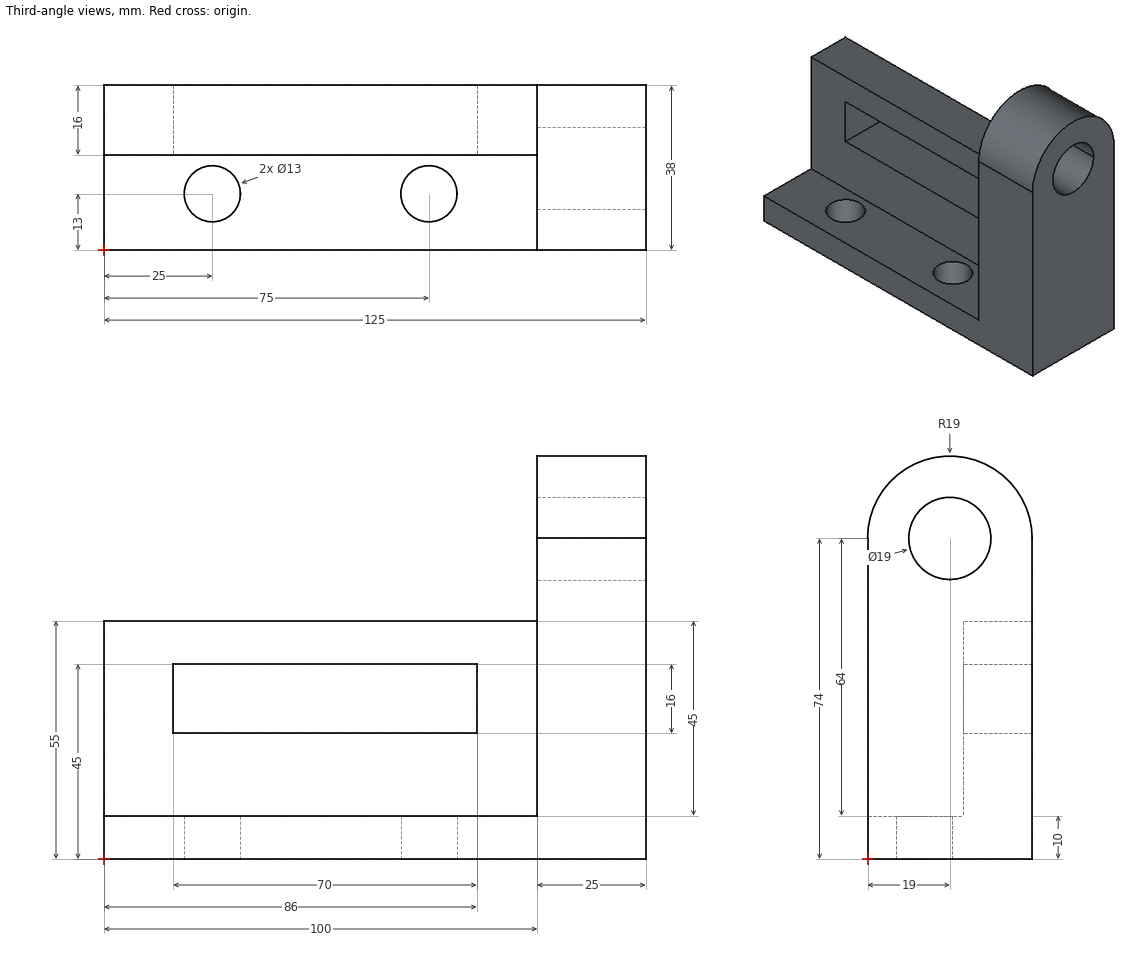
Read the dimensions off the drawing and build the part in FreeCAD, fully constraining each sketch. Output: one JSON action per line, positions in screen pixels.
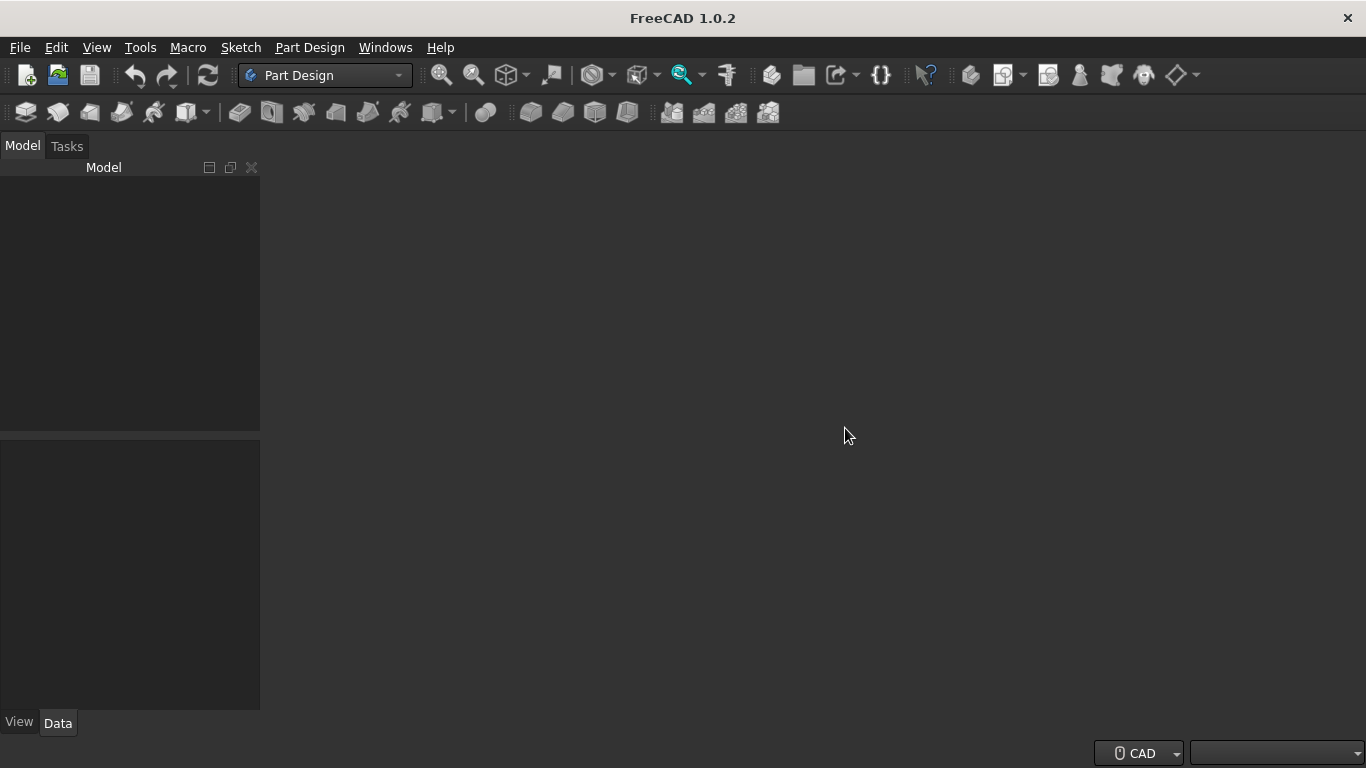
{"action": "left_click", "coordinate": [26, 76]}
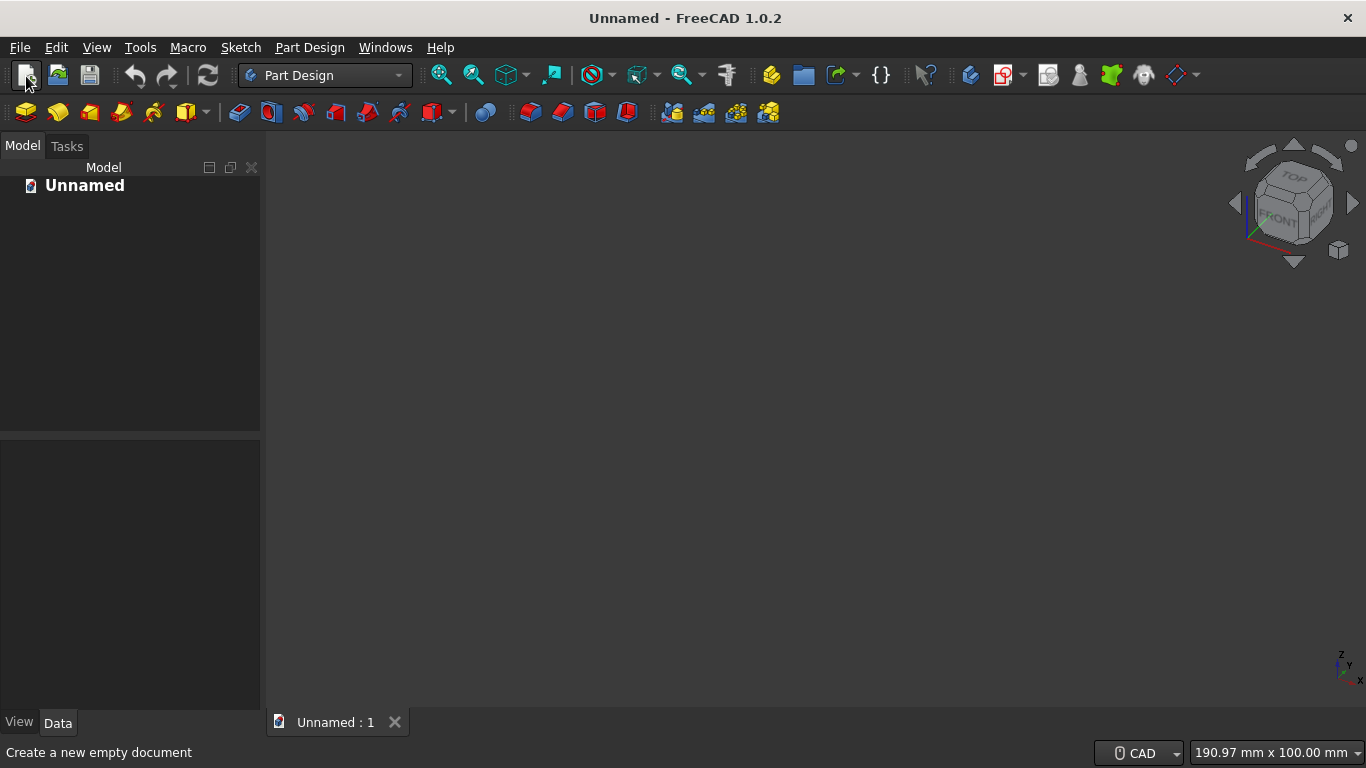
{"action": "left_click", "coordinate": [1004, 76]}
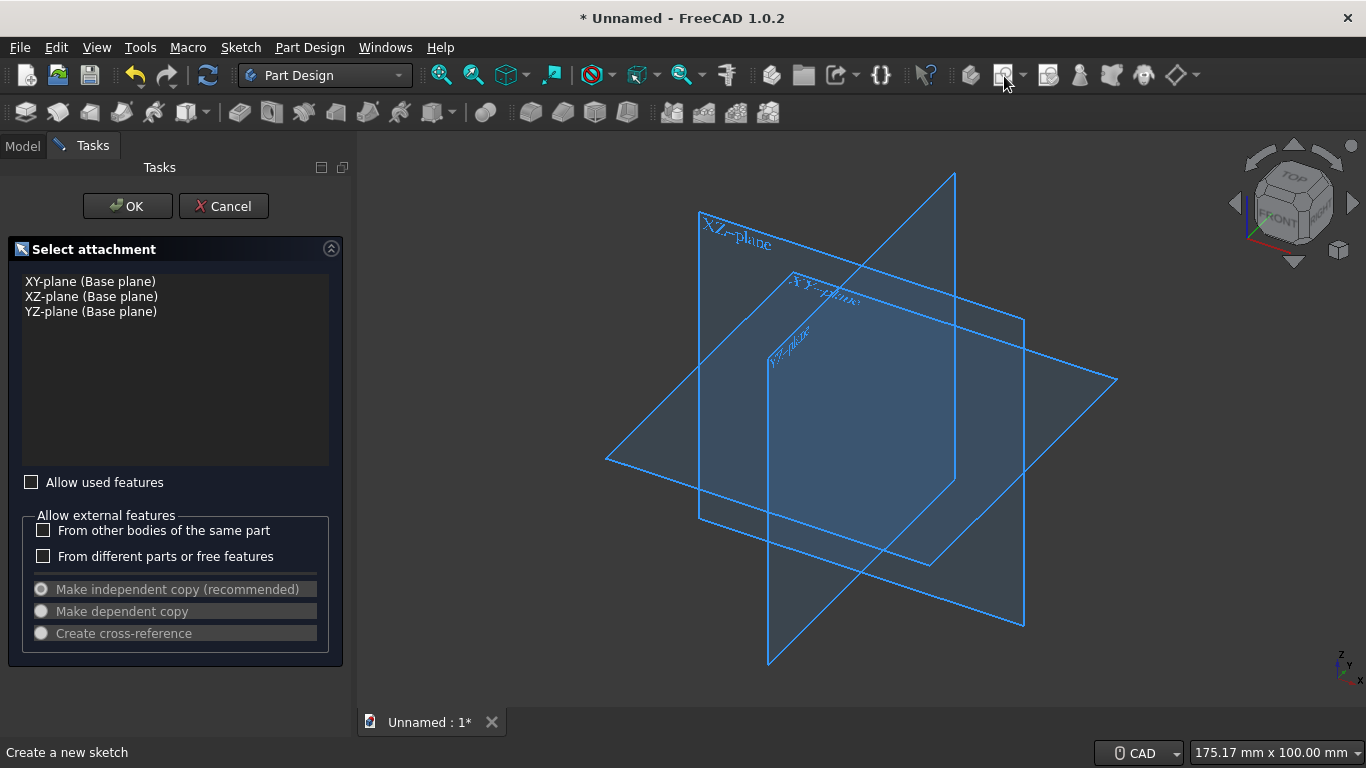
{"action": "left_click", "coordinate": [82, 282]}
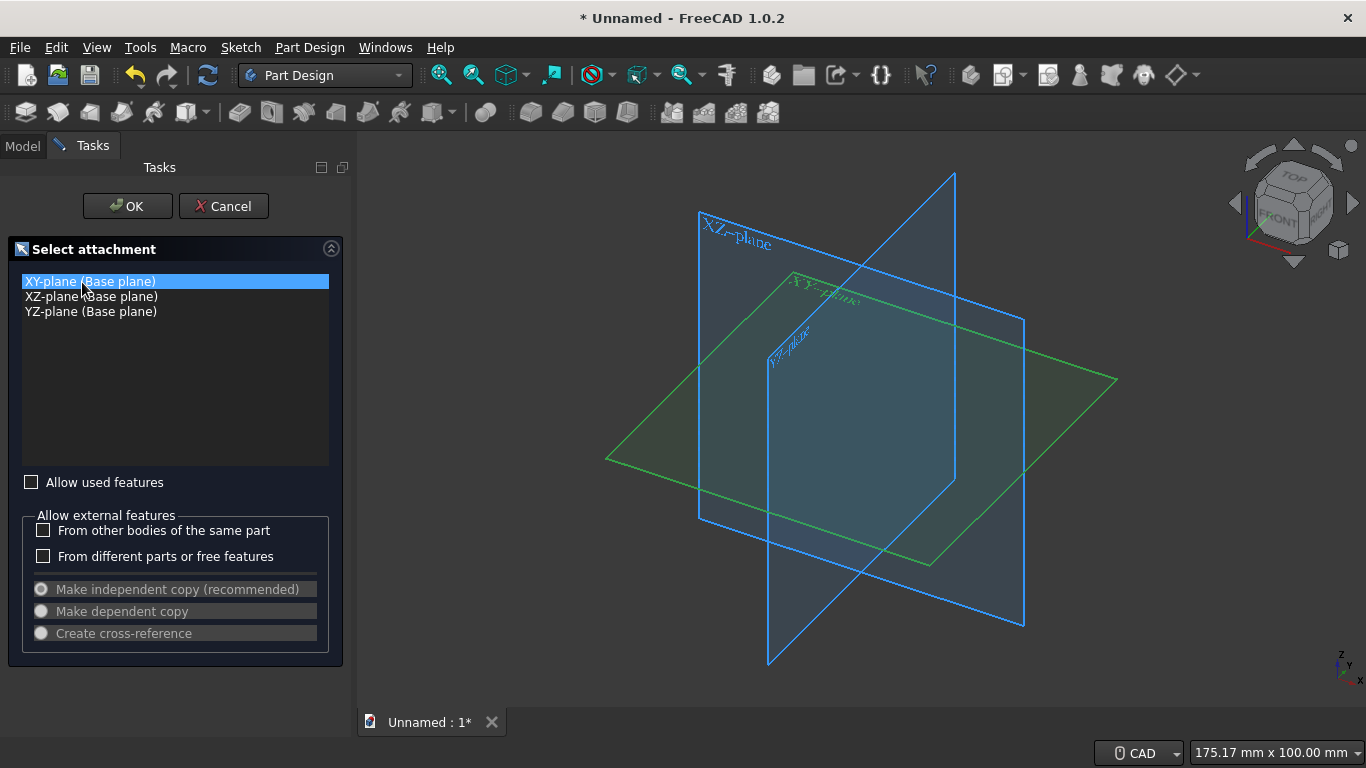
{"action": "left_click", "coordinate": [128, 206]}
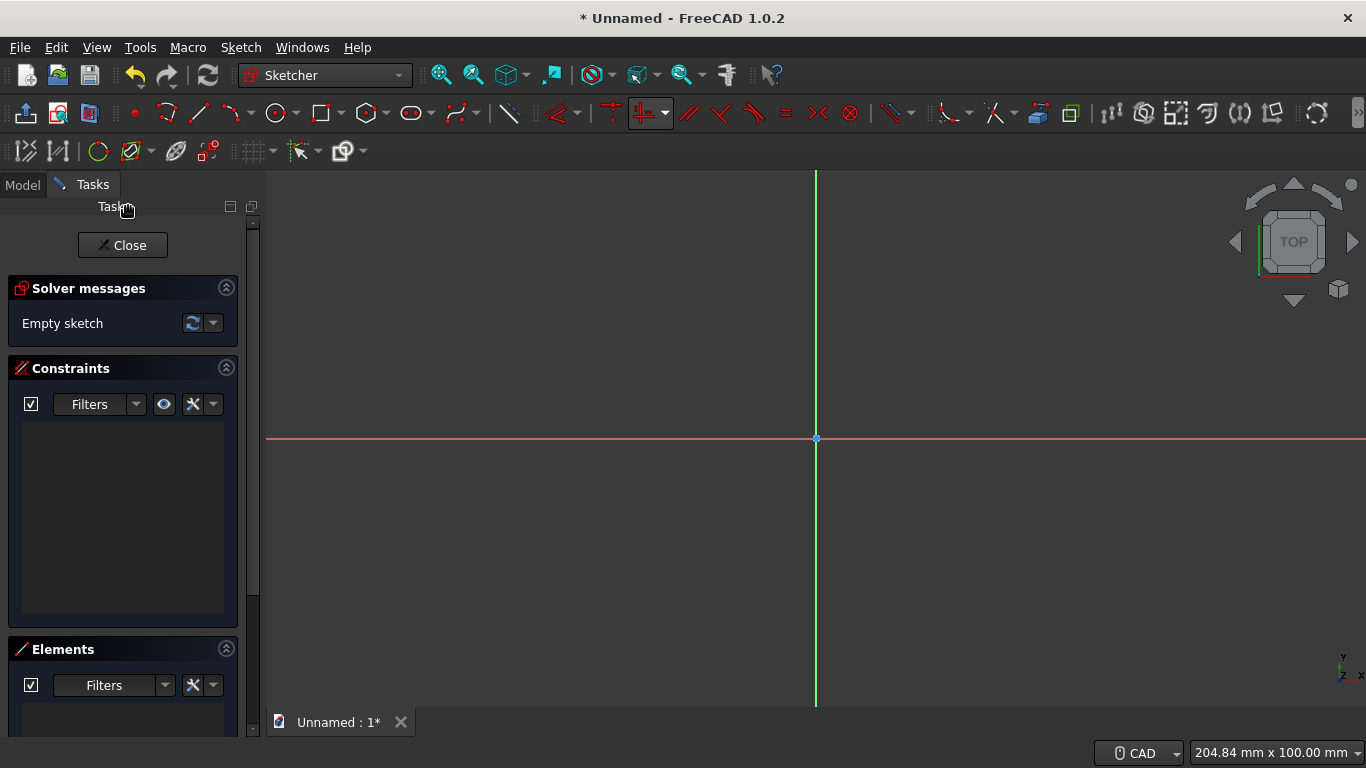
{"action": "scroll", "coordinate": [294, 646], "scroll_direction": "down", "scroll_amount": 2}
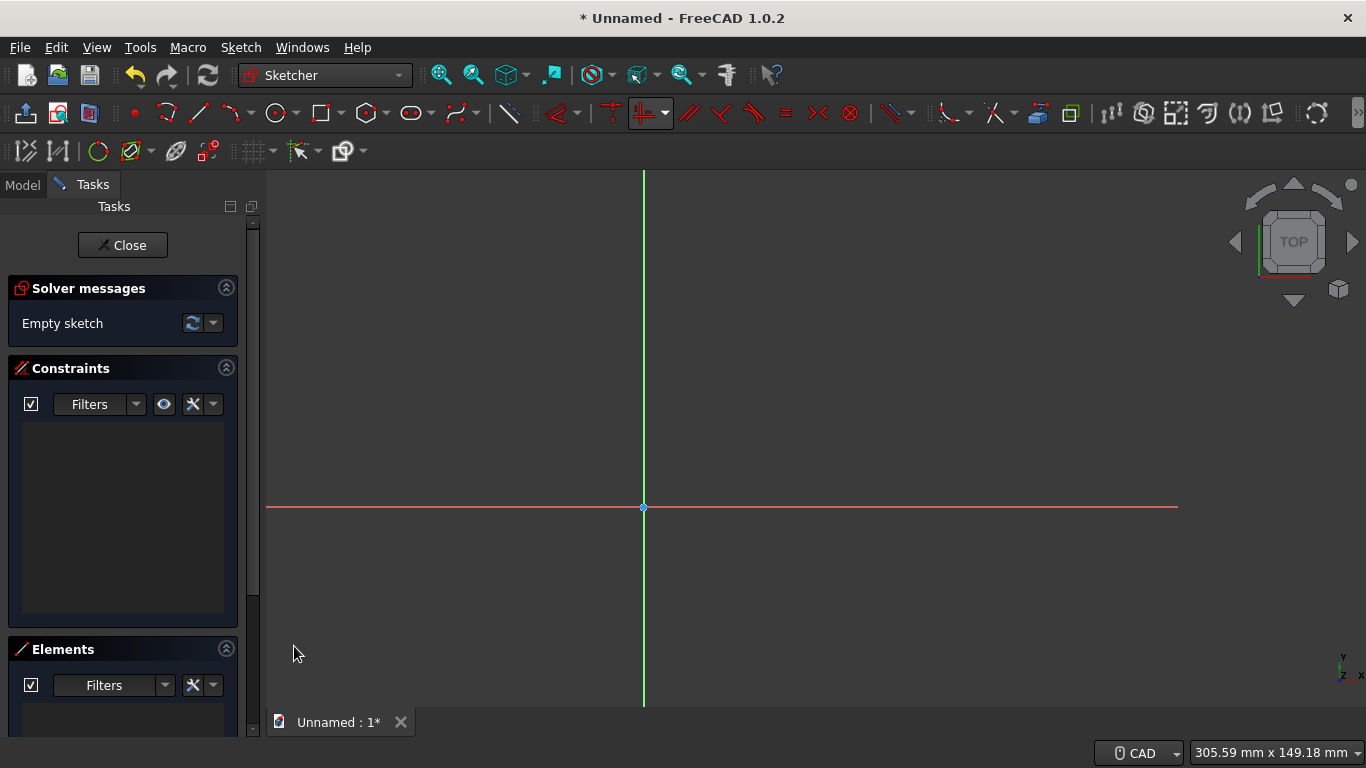
{"action": "scroll", "coordinate": [1116, 439], "scroll_direction": "up", "scroll_amount": 2}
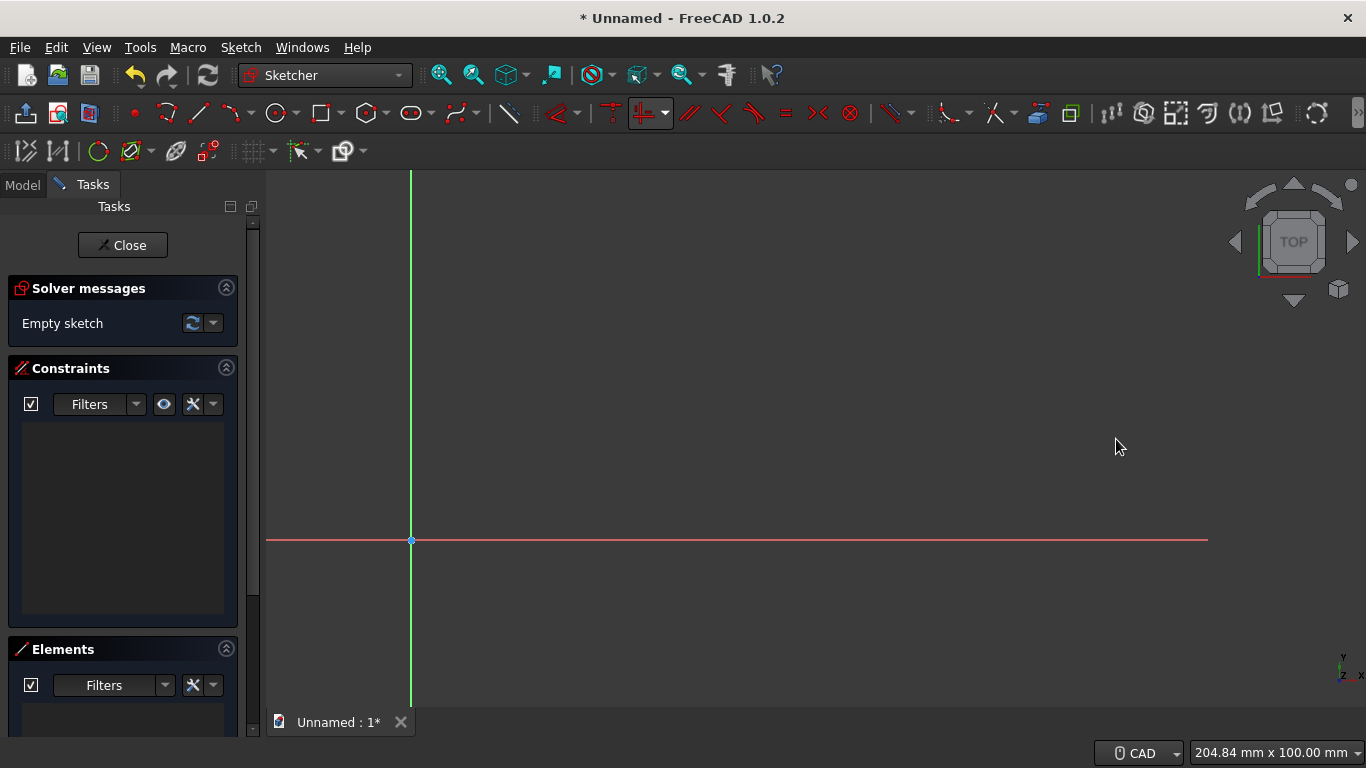
{"action": "left_click", "coordinate": [322, 114]}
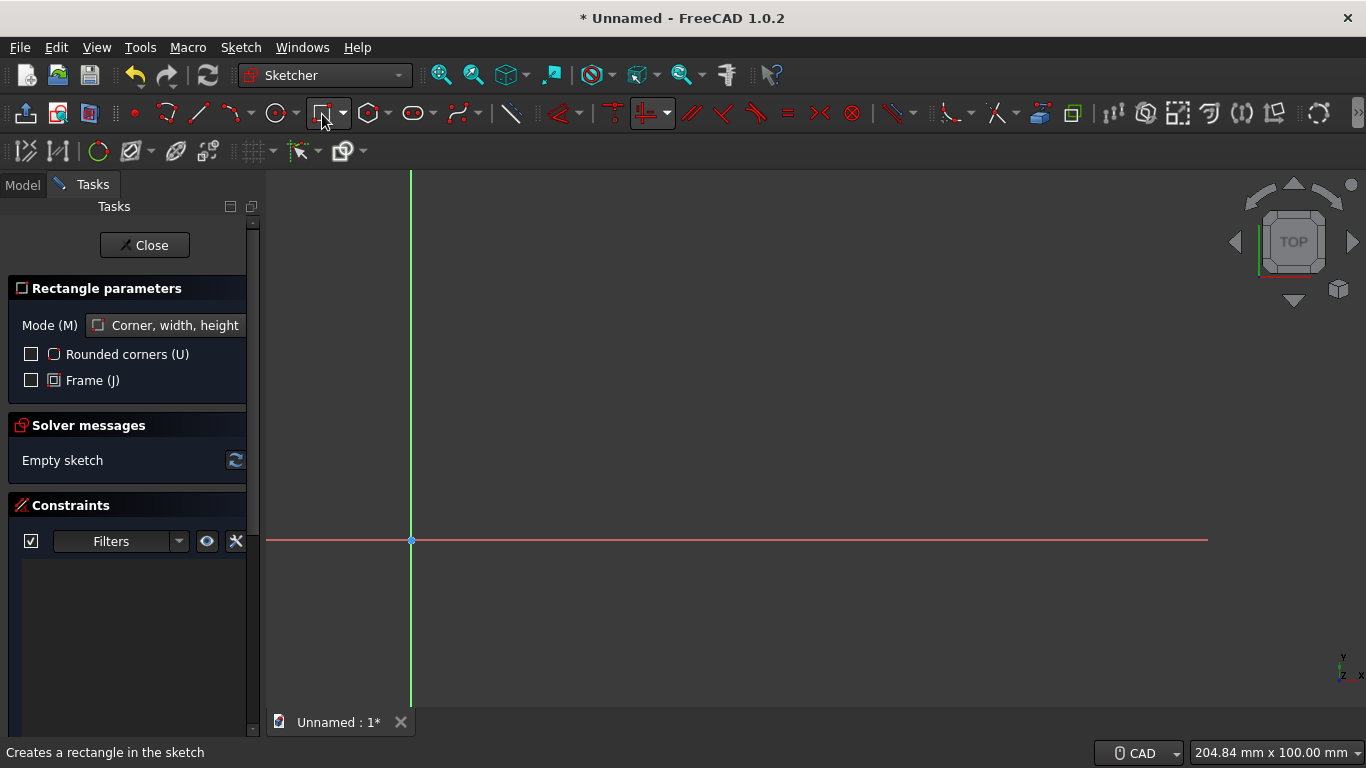
{"action": "left_click", "coordinate": [411, 540]}
{"action": "left_click", "coordinate": [1083, 336]}
{"action": "key", "text": "Escape"}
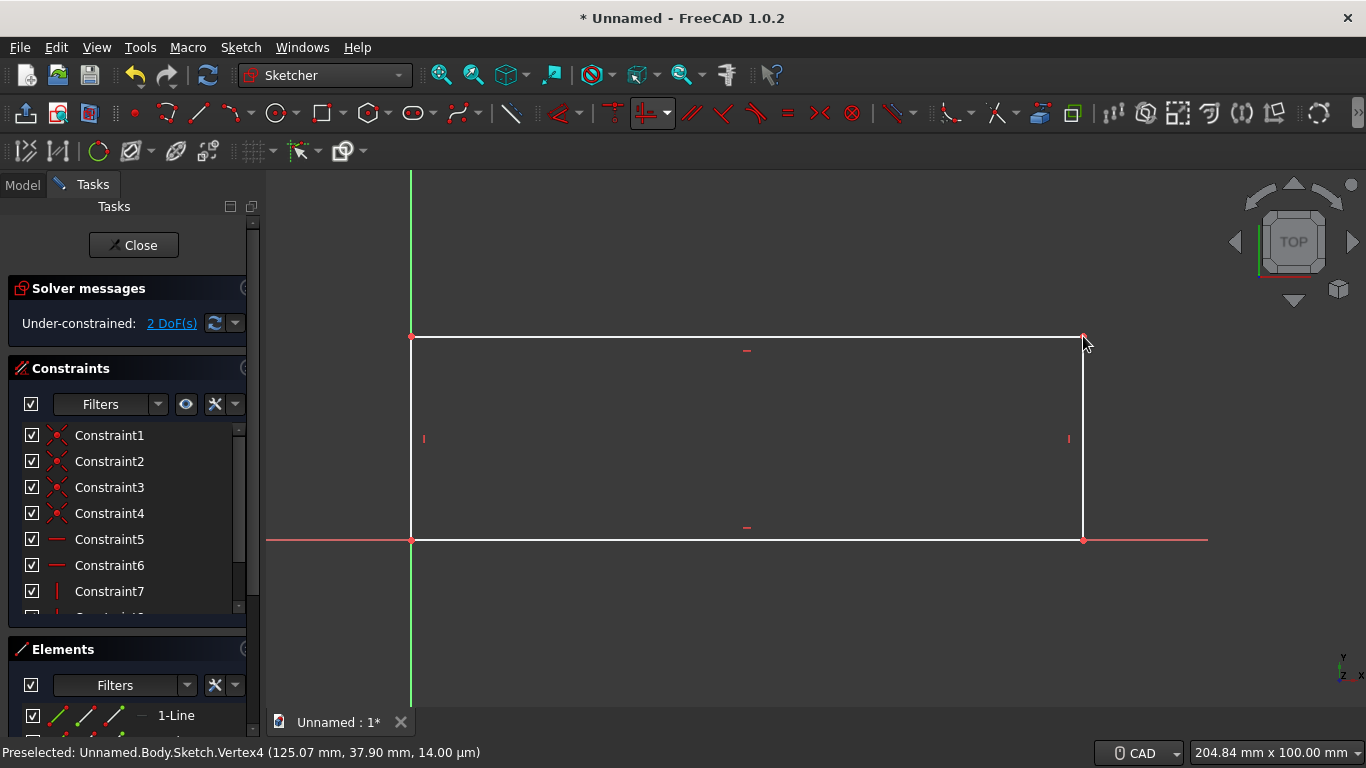
{"action": "left_click", "coordinate": [558, 114]}